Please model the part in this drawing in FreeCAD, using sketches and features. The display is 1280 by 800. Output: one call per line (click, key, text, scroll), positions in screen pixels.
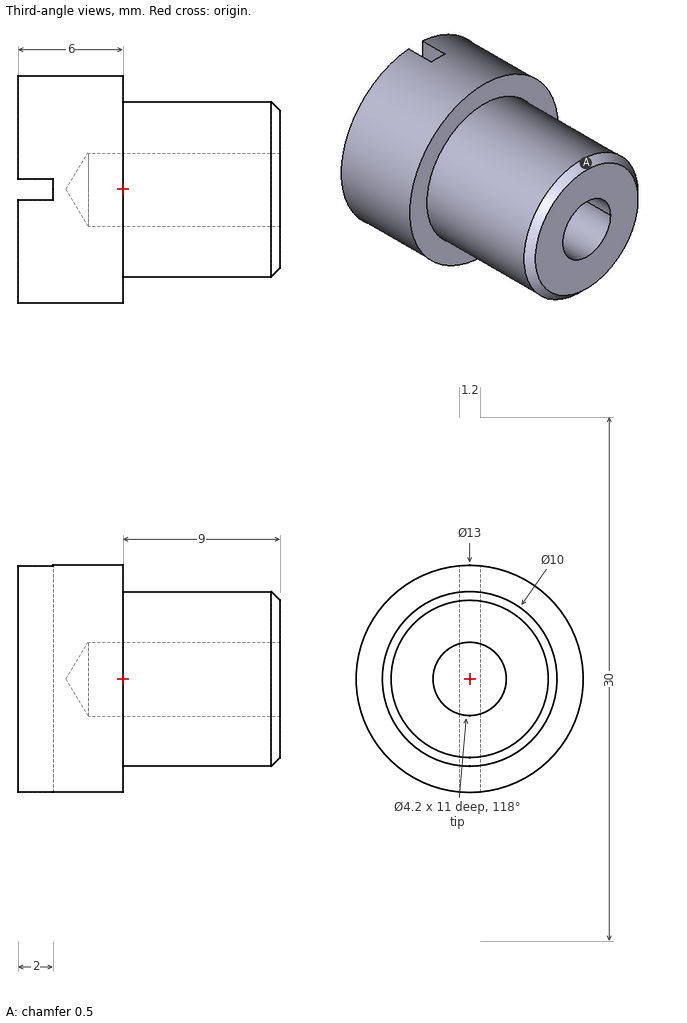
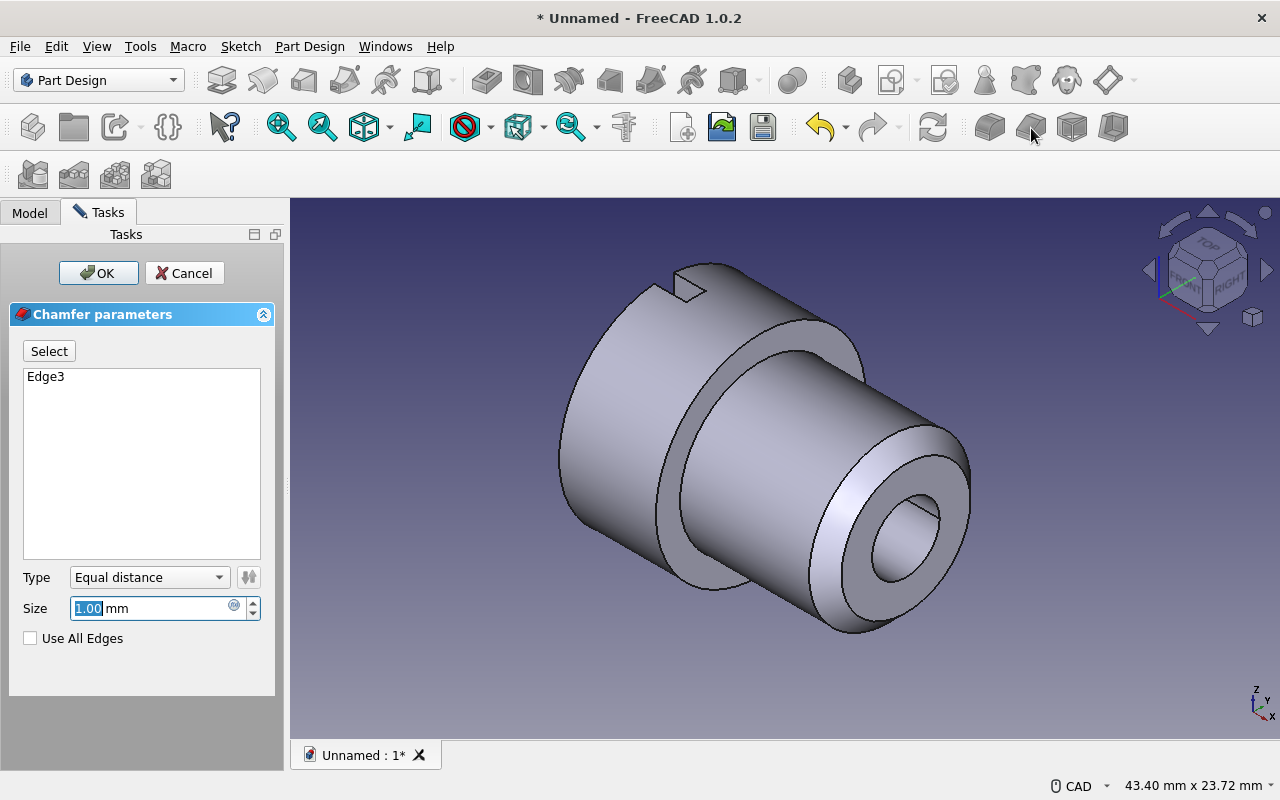
text(0.5)
key(Tab)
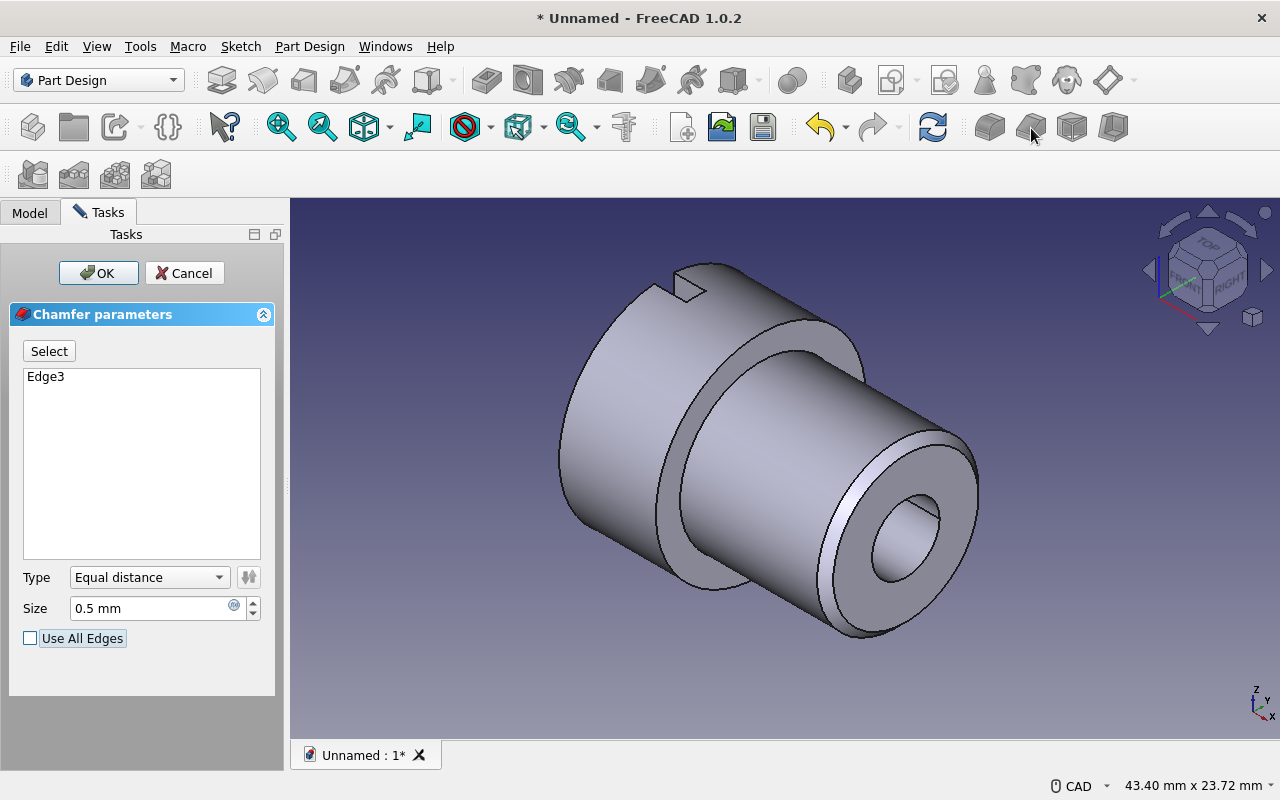
click(99, 273)